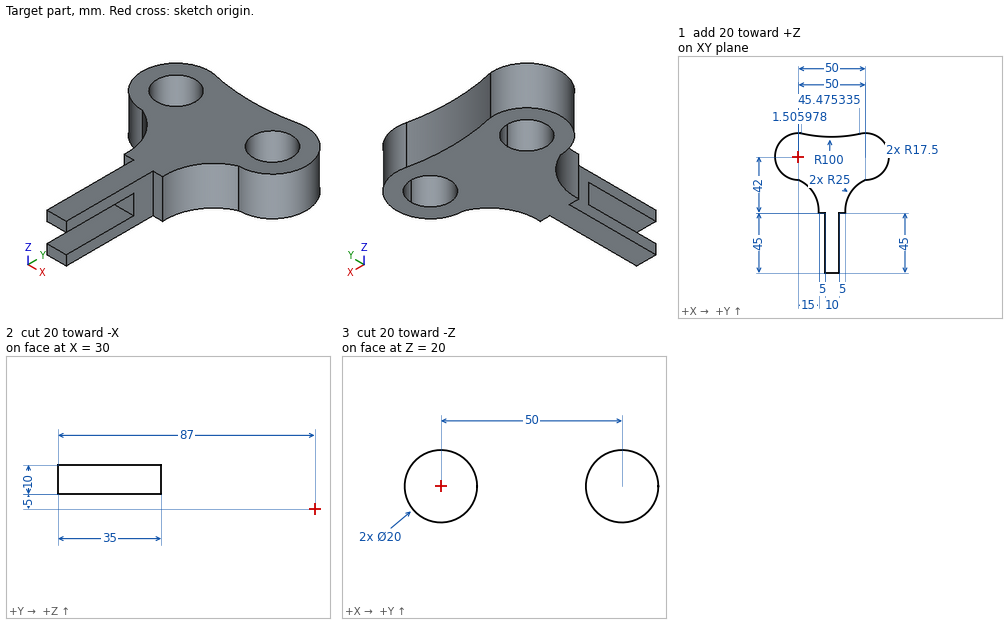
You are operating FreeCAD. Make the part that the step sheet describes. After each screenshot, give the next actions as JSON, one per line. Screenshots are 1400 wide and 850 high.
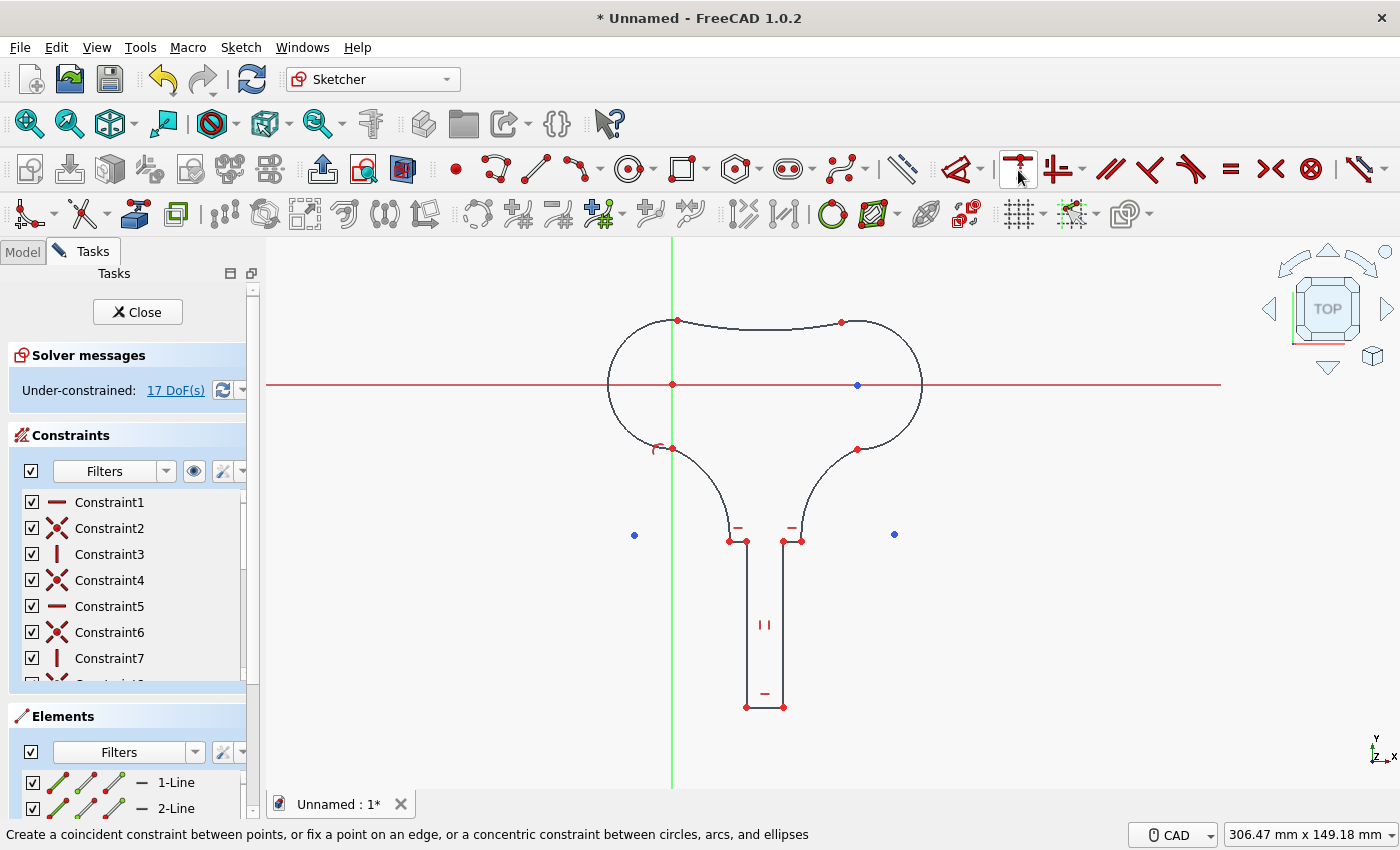
{"action": "left_click", "coordinate": [912, 419]}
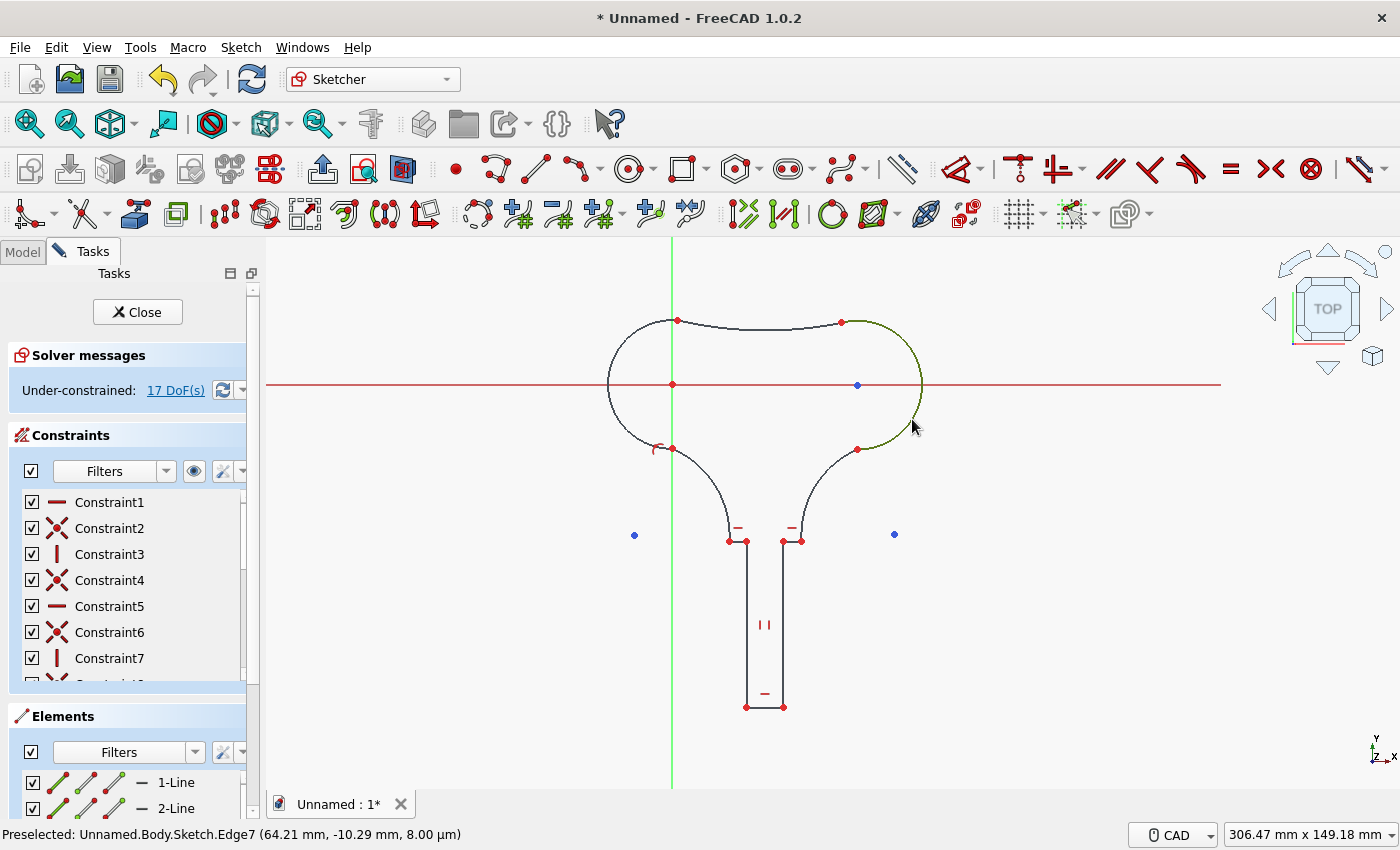
{"action": "left_click", "coordinate": [623, 344]}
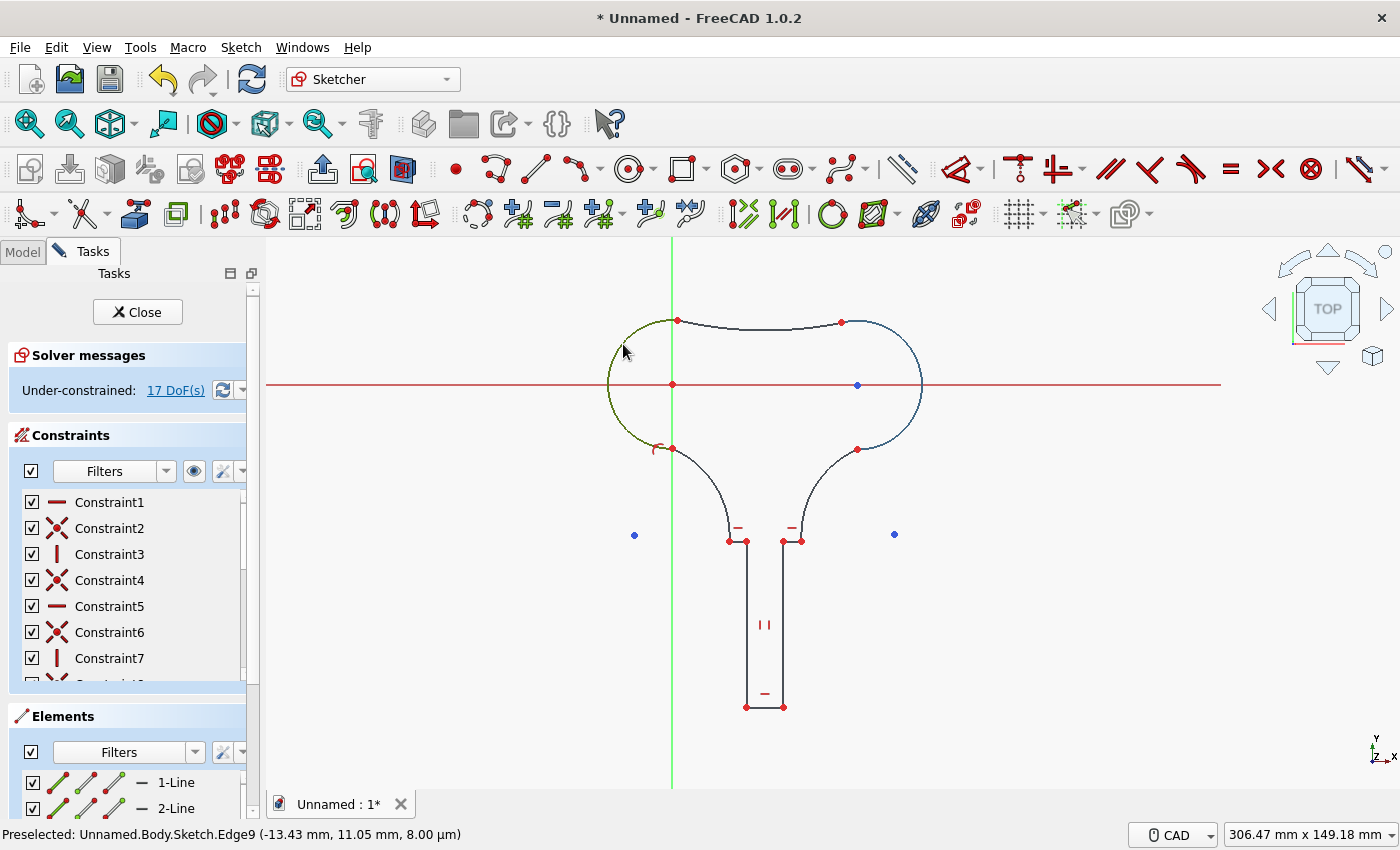
{"action": "left_click", "coordinate": [1232, 170]}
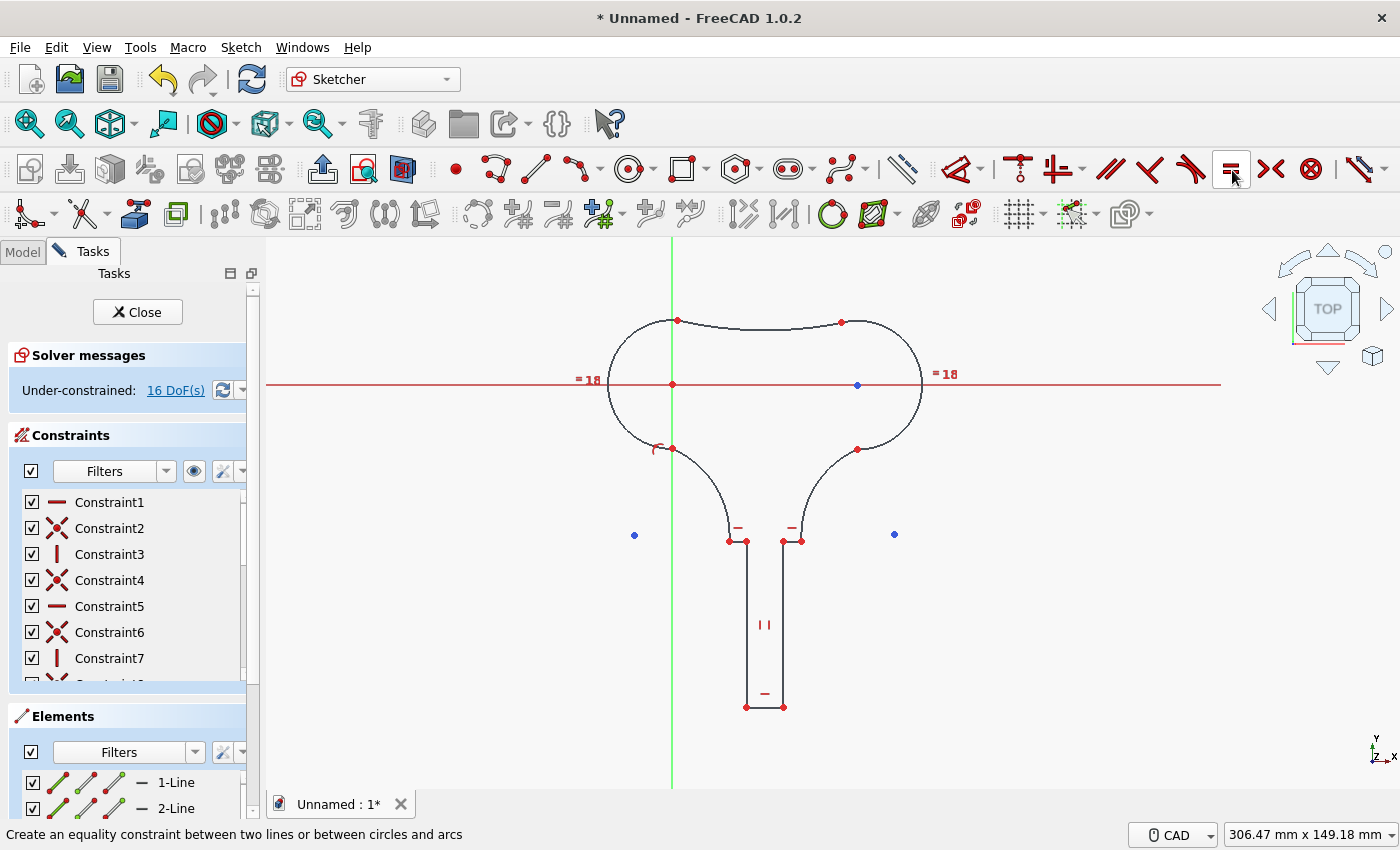
{"action": "left_click", "coordinate": [829, 469]}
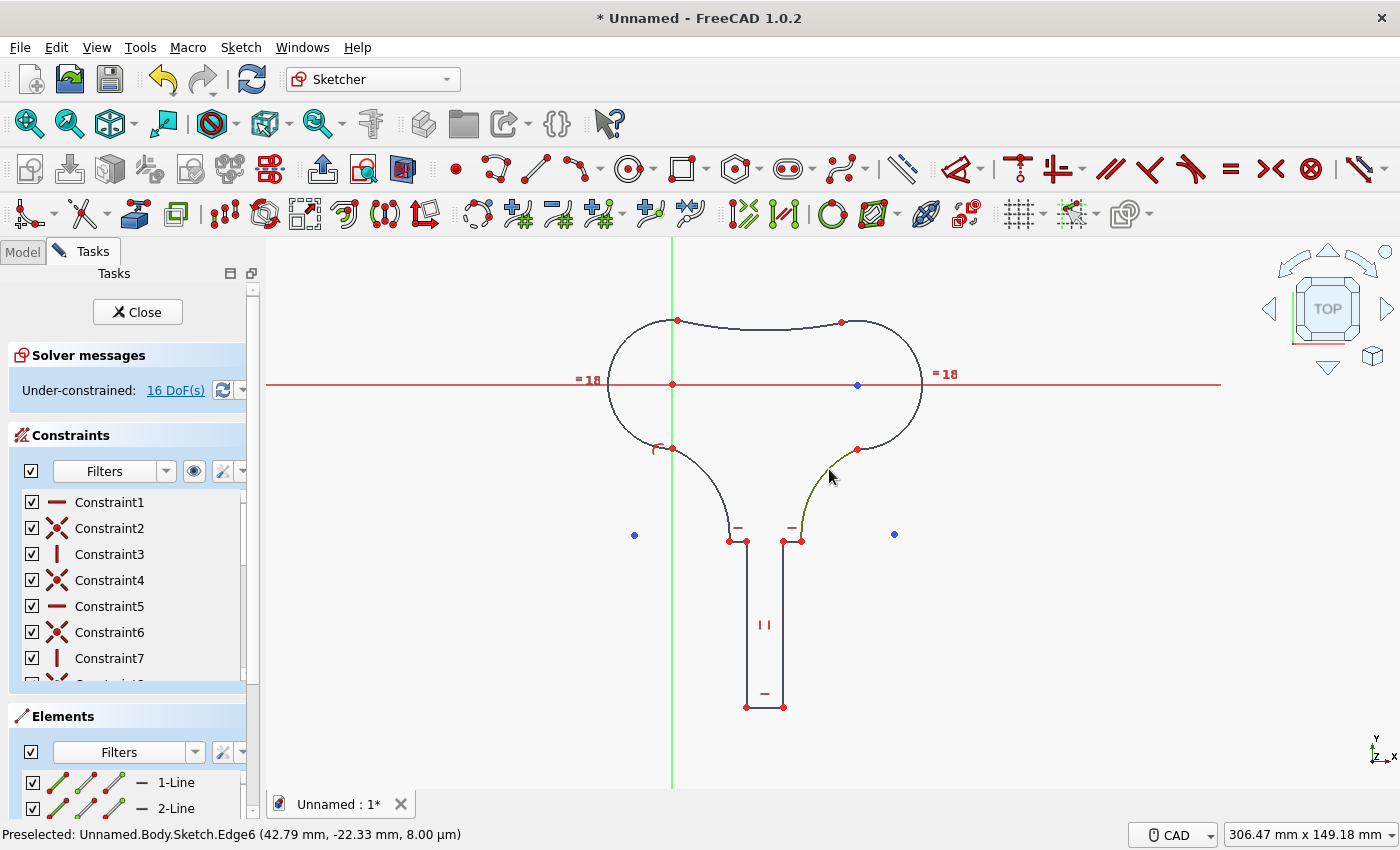
{"action": "left_click", "coordinate": [725, 507]}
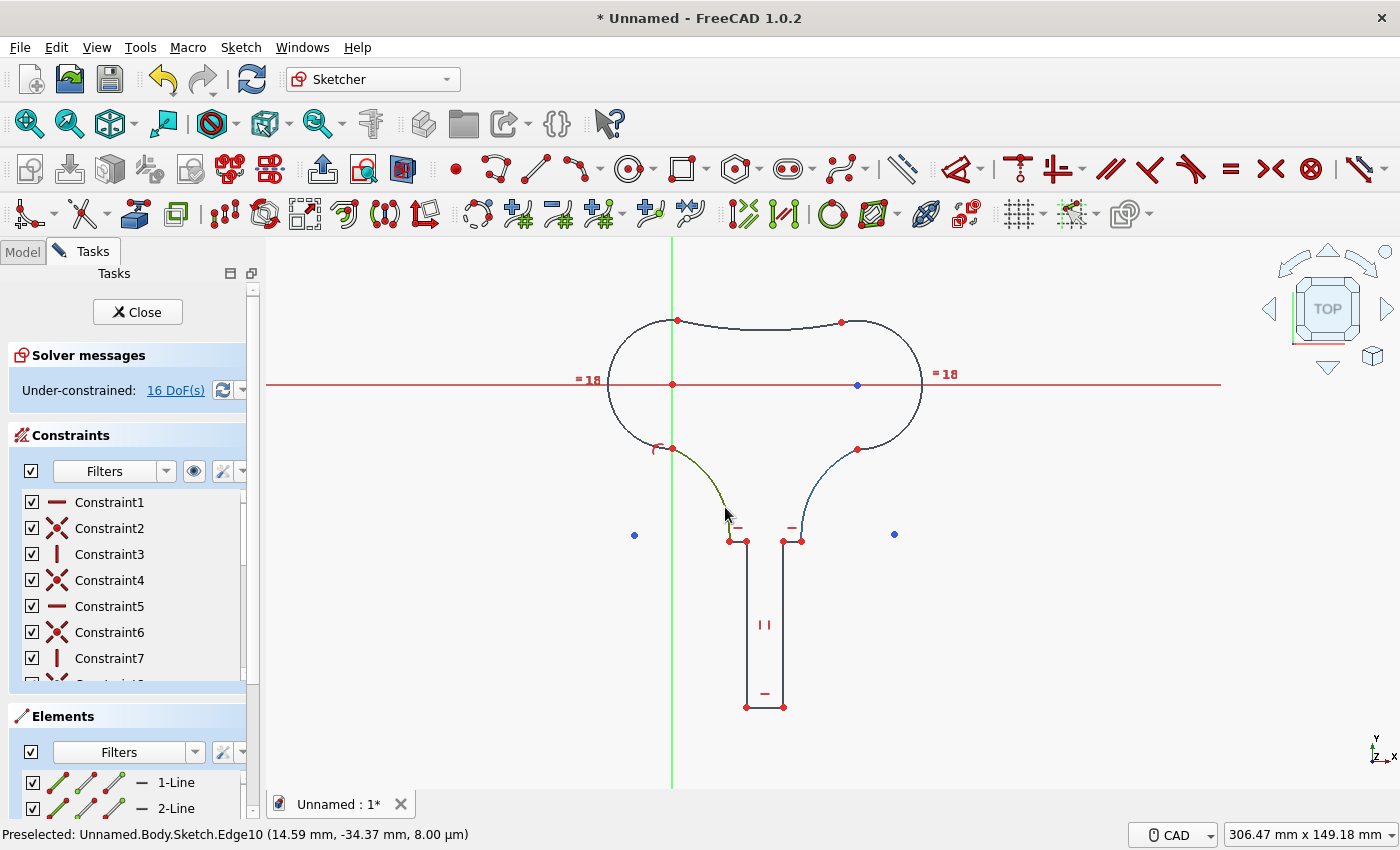
{"action": "left_click", "coordinate": [1232, 170]}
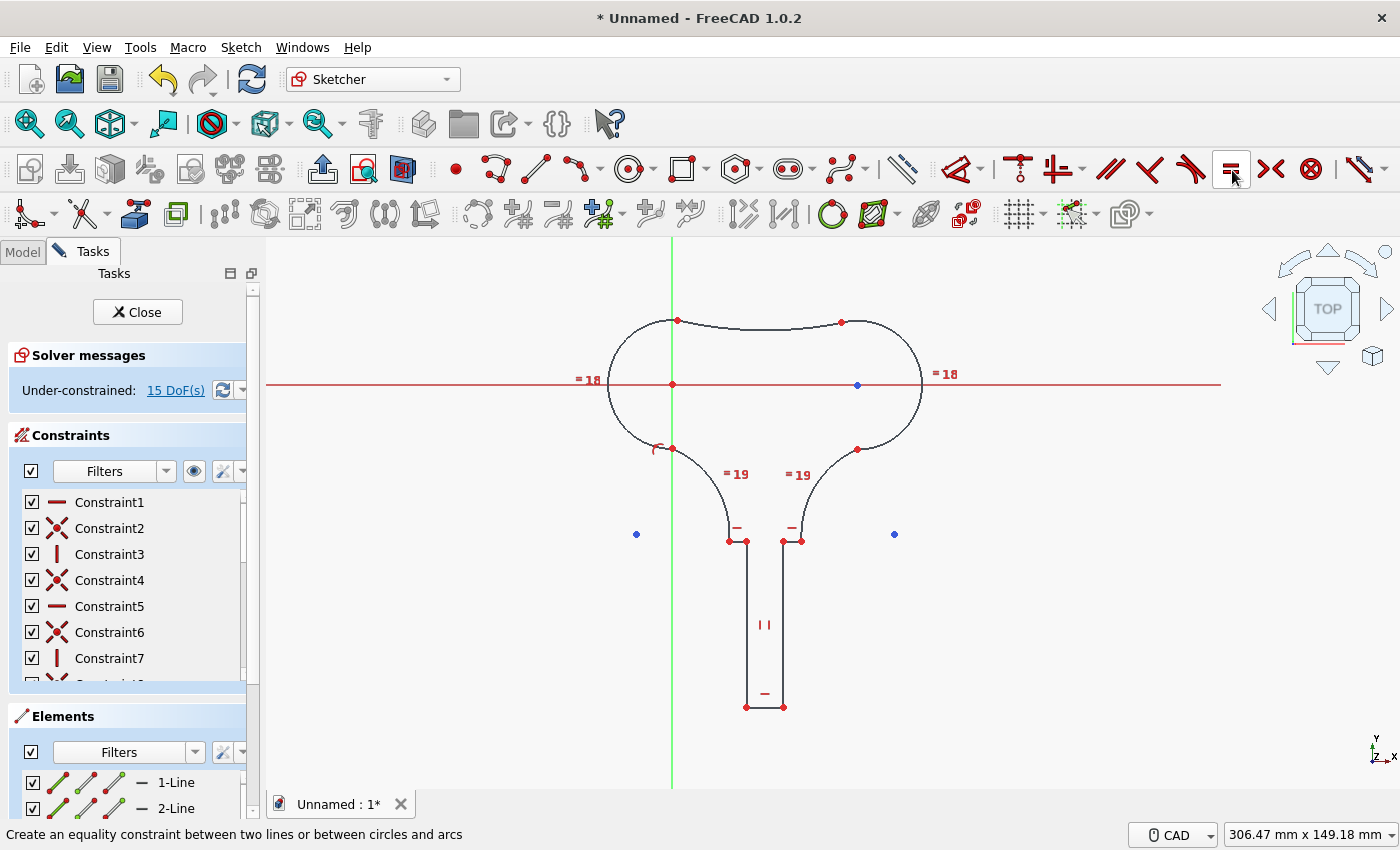
{"action": "left_click", "coordinate": [858, 385]}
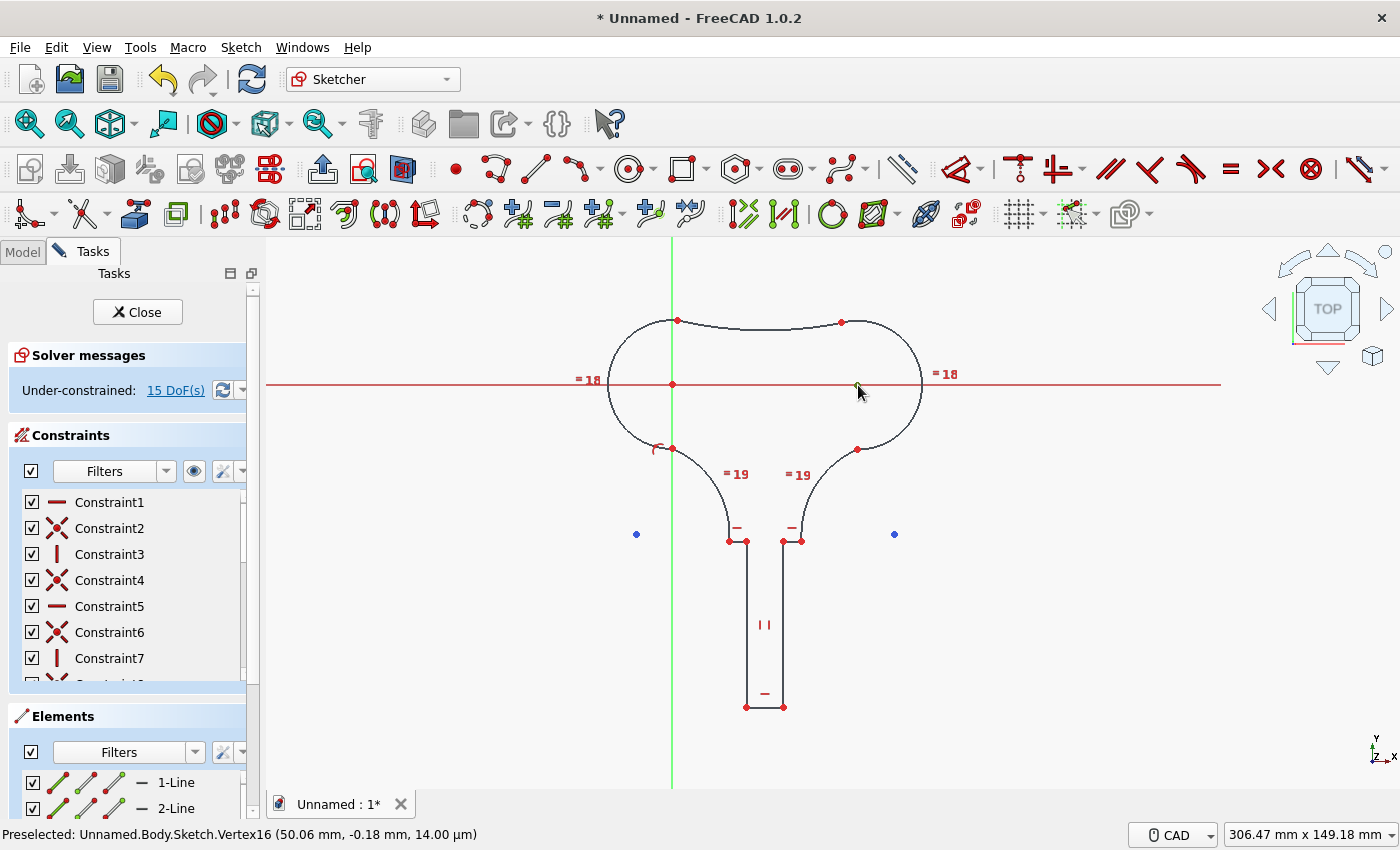
{"action": "left_click", "coordinate": [361, 385]}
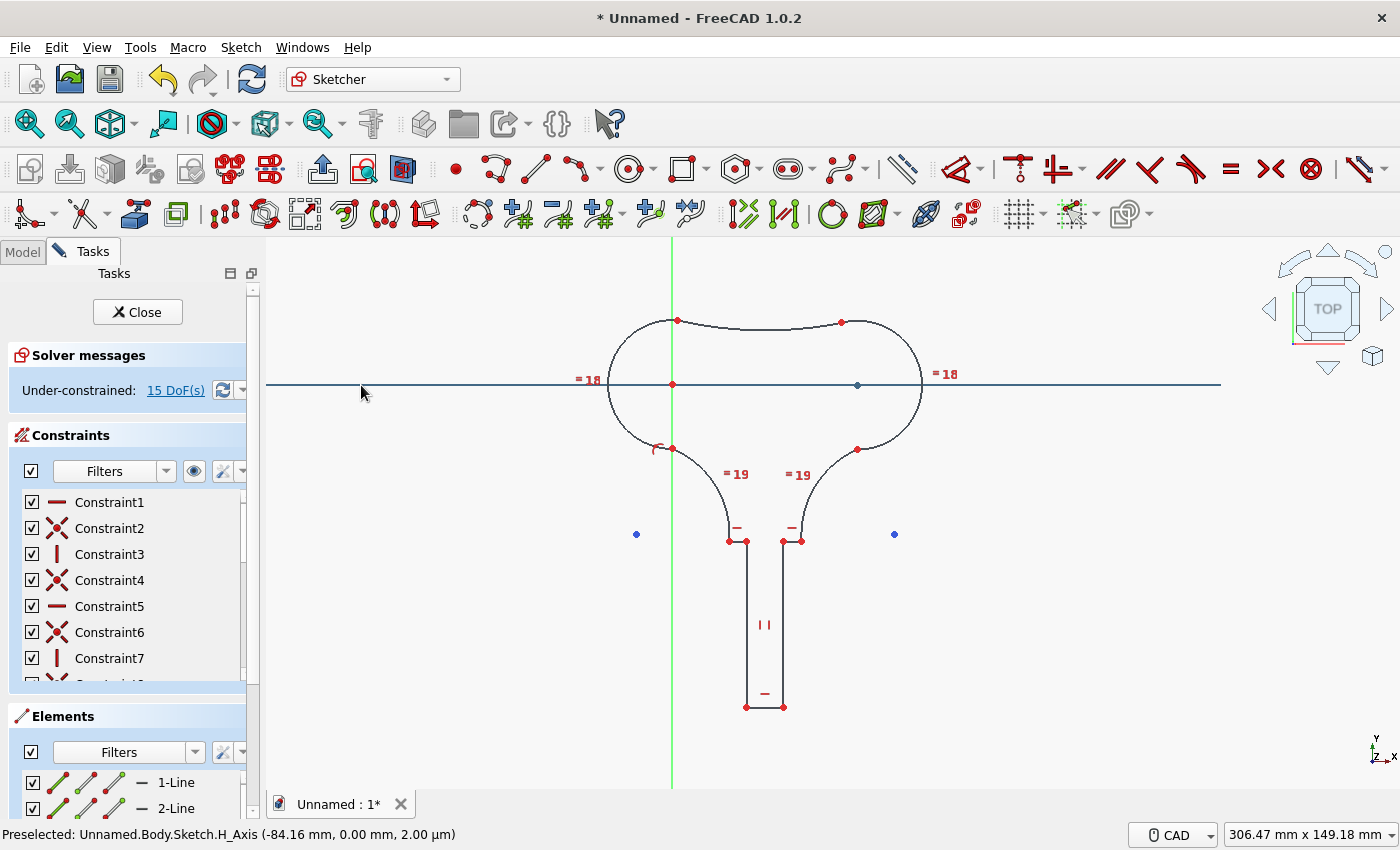
{"action": "left_click", "coordinate": [1018, 170]}